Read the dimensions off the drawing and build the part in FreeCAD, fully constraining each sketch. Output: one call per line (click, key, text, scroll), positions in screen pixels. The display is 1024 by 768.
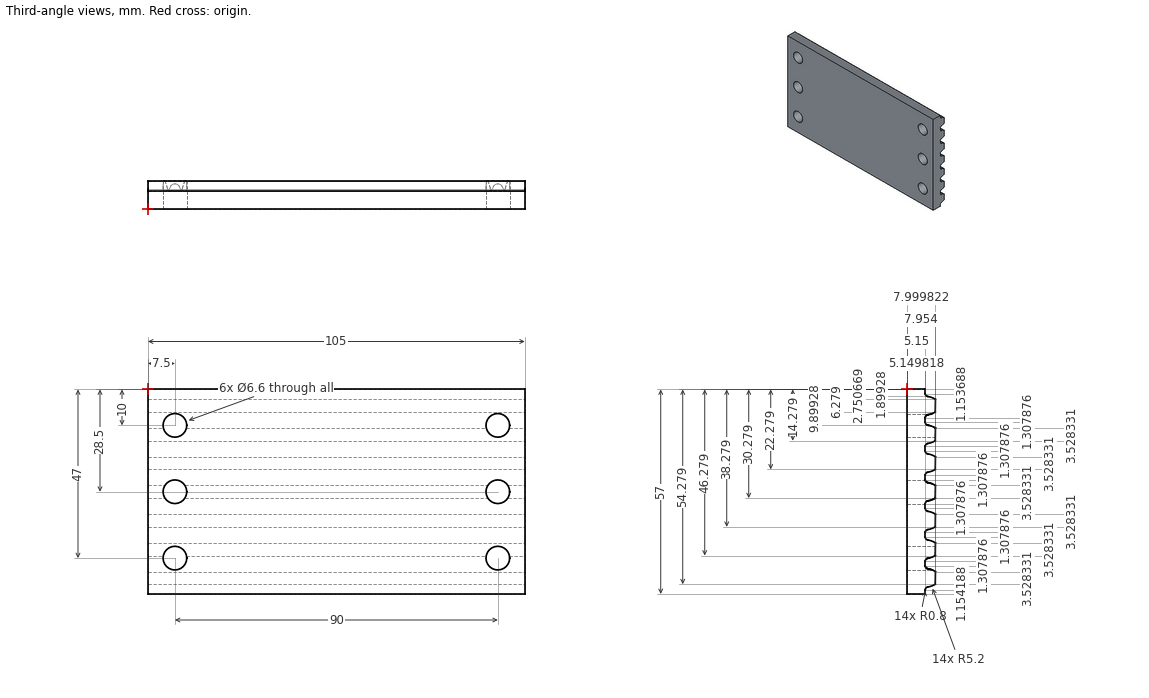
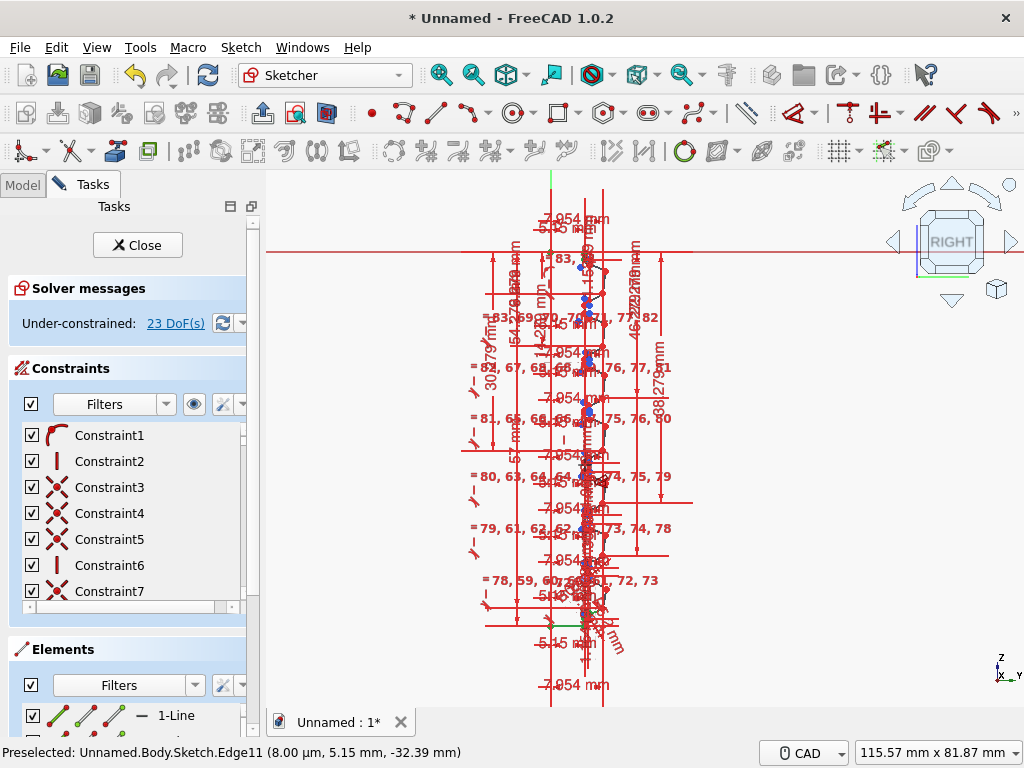
scroll(585, 413, up, 13)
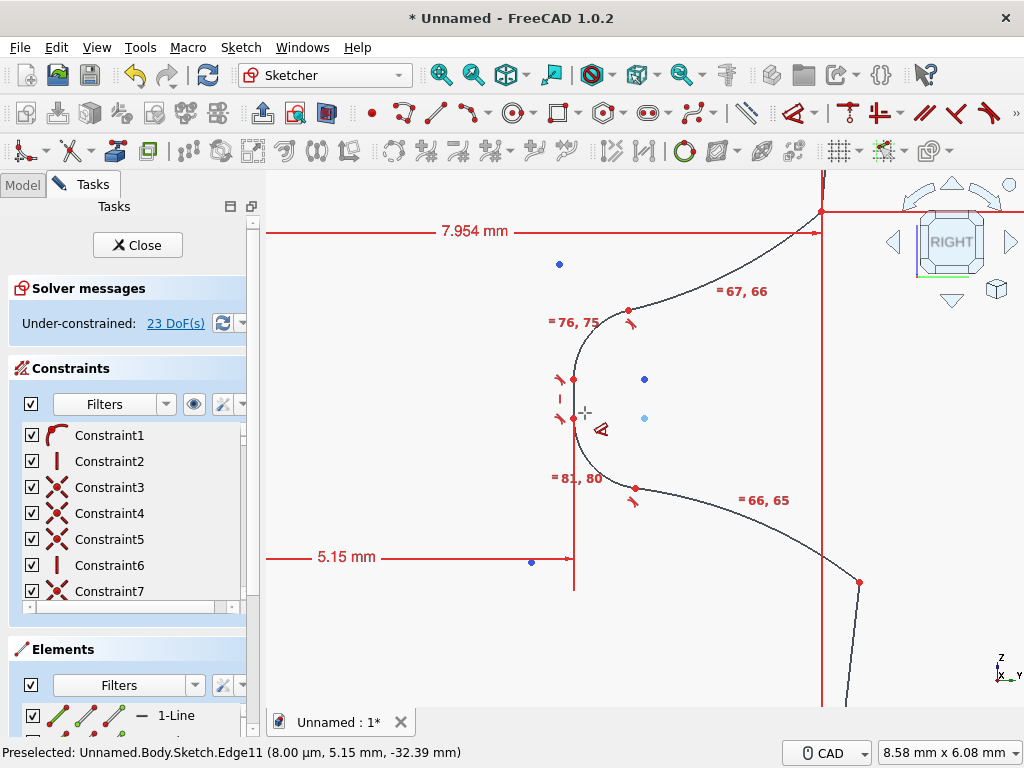
click(574, 403)
click(608, 399)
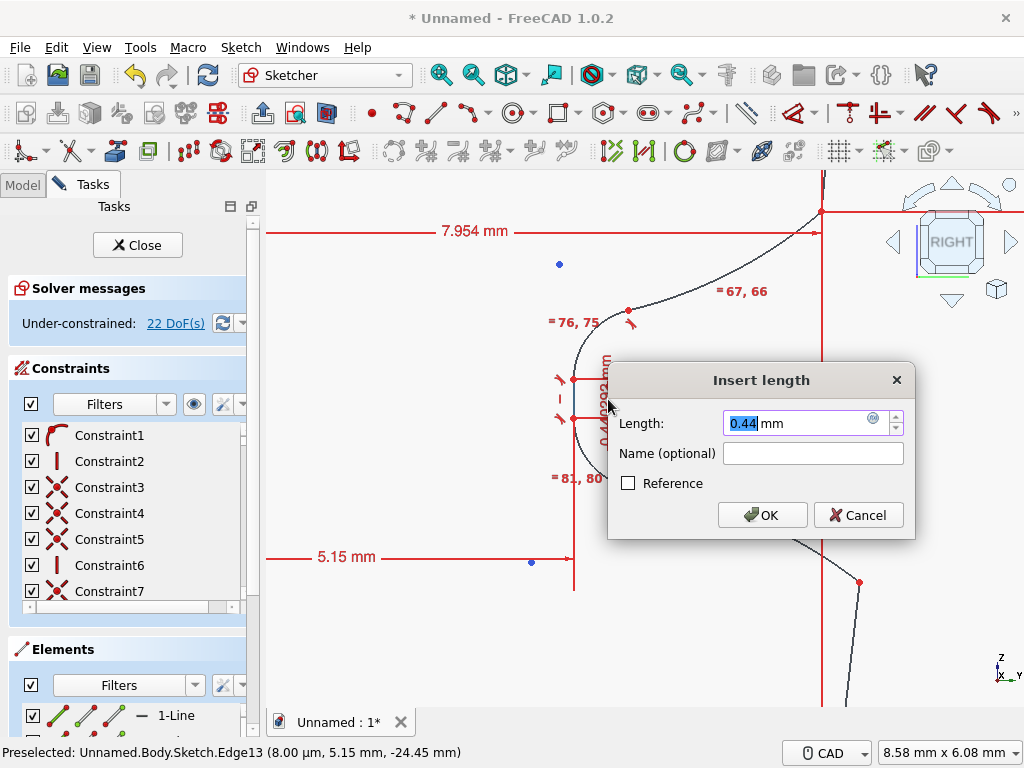
text(1.307876)
key(Return)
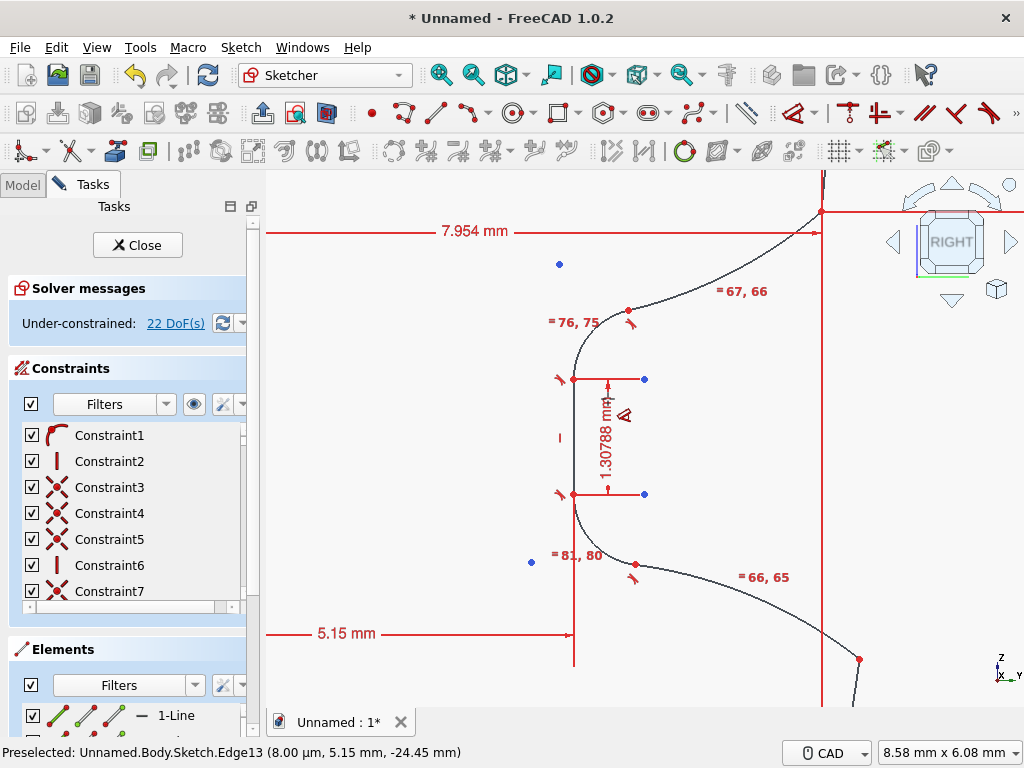
scroll(585, 413, down, 13)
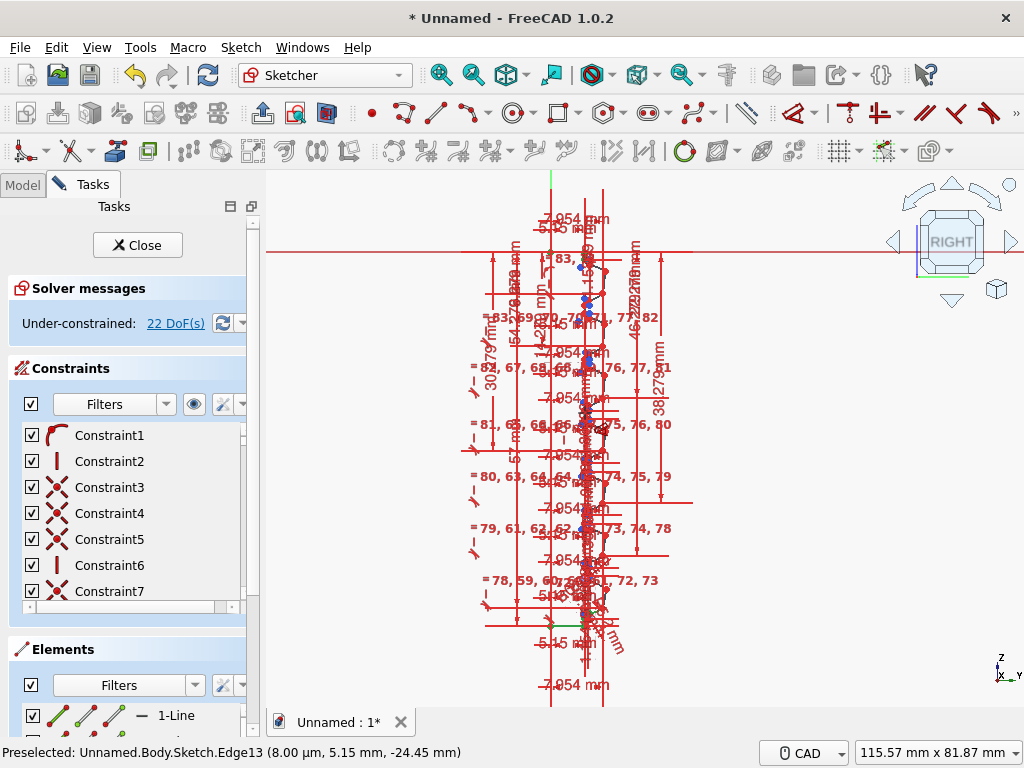
scroll(585, 362, up, 13)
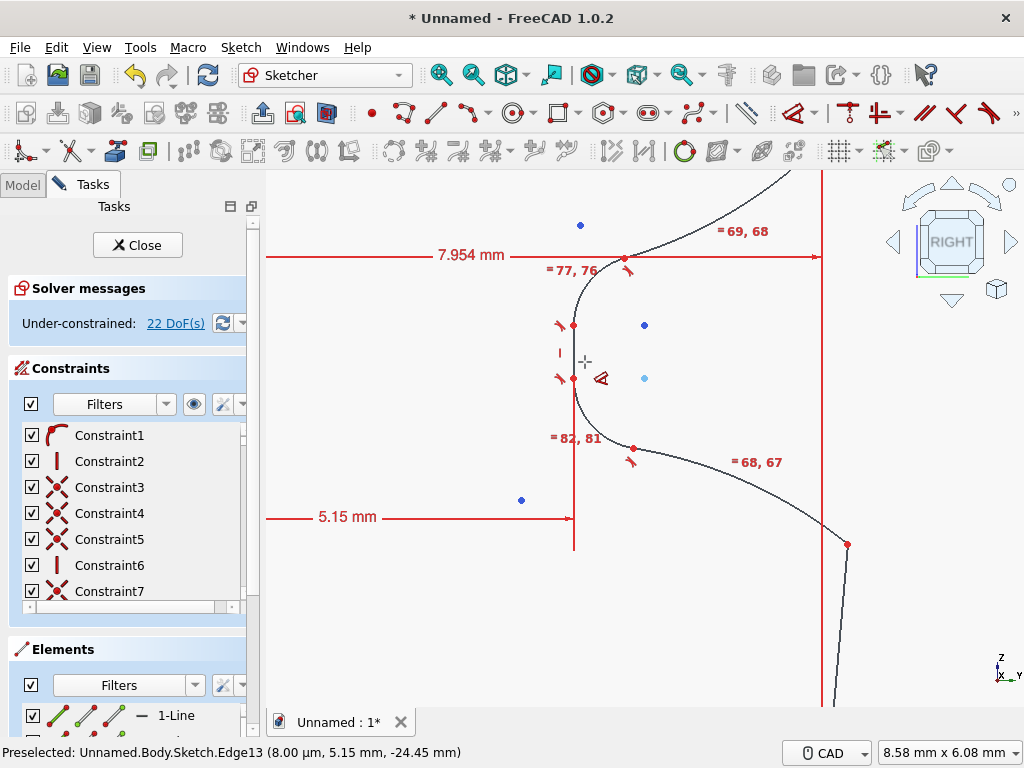
click(574, 363)
click(608, 352)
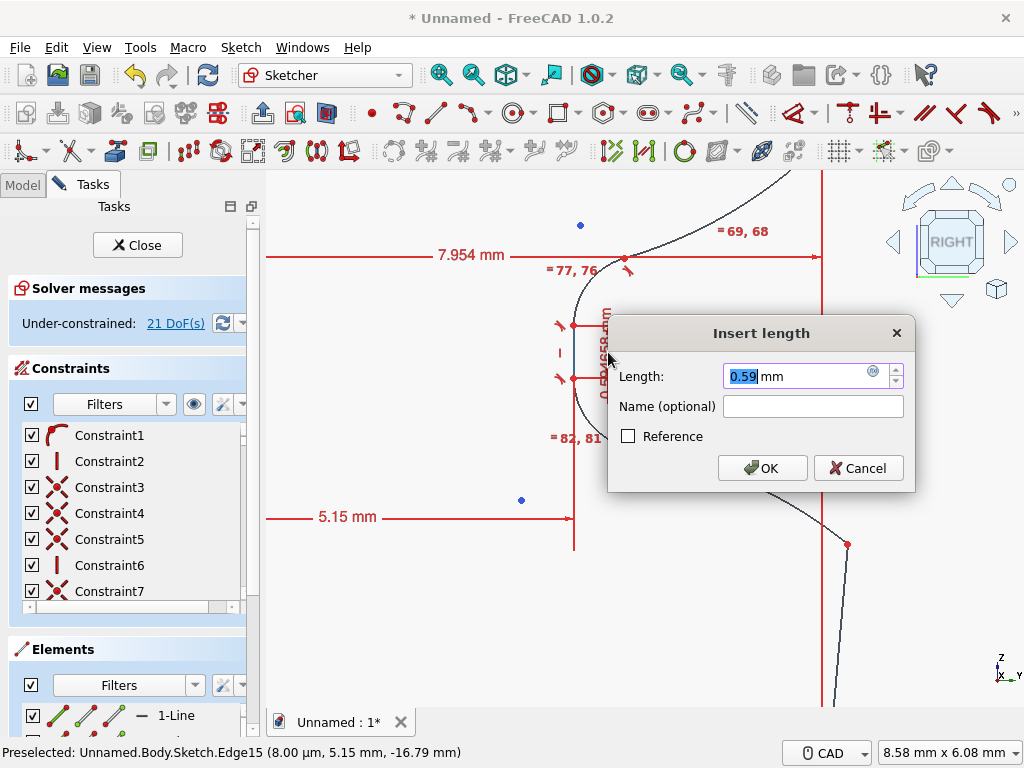
text(1.307876)
key(Return)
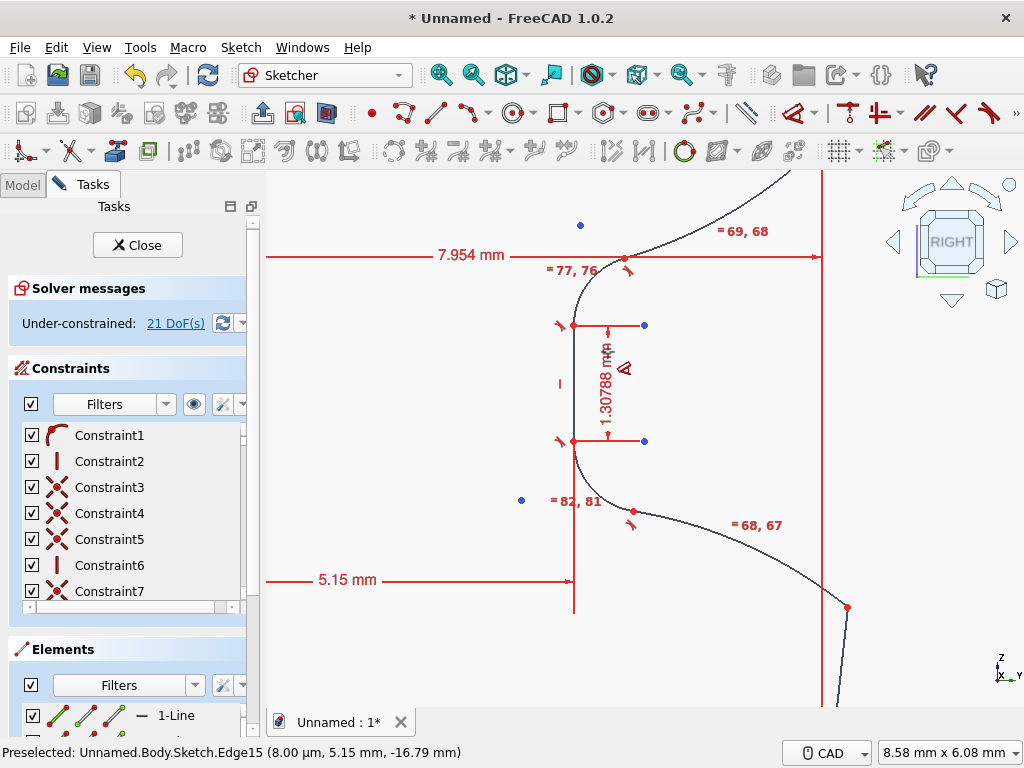
scroll(585, 362, down, 13)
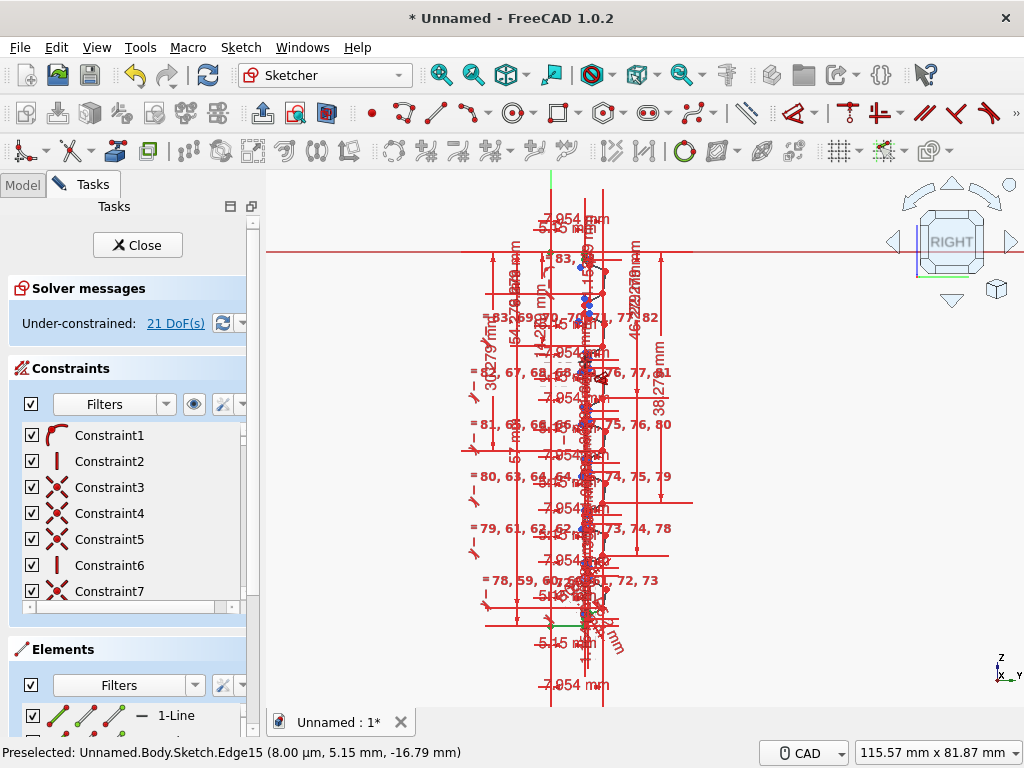
scroll(585, 311, up, 10)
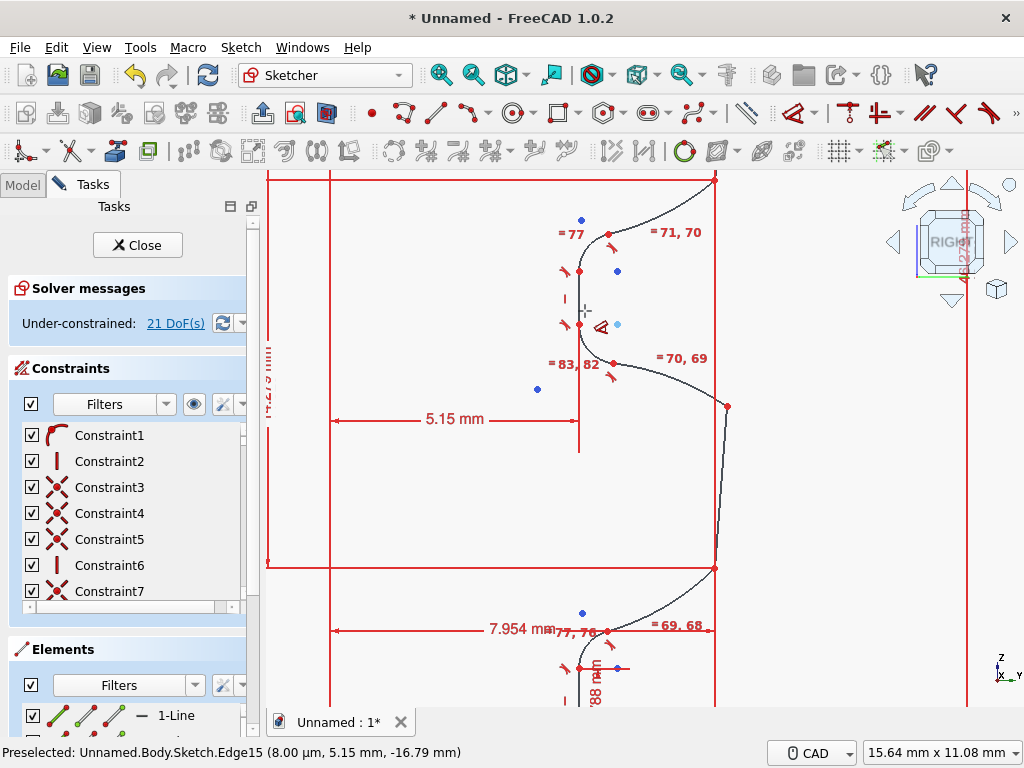
click(579, 309)
click(613, 298)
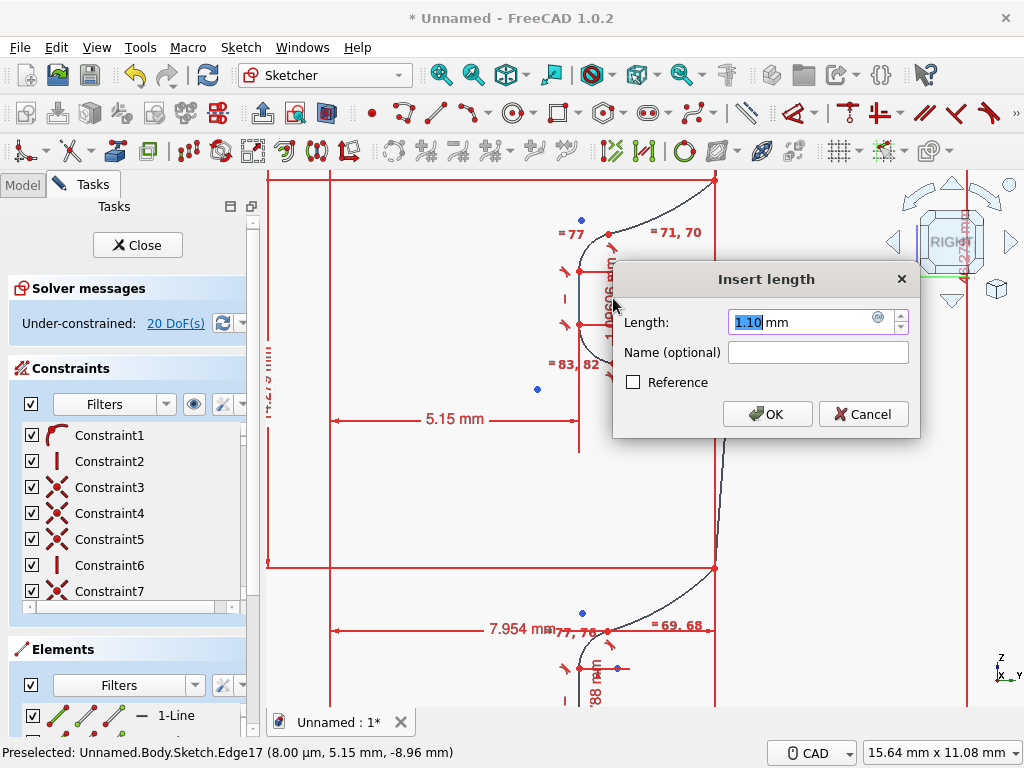
text(1.307876)
key(Return)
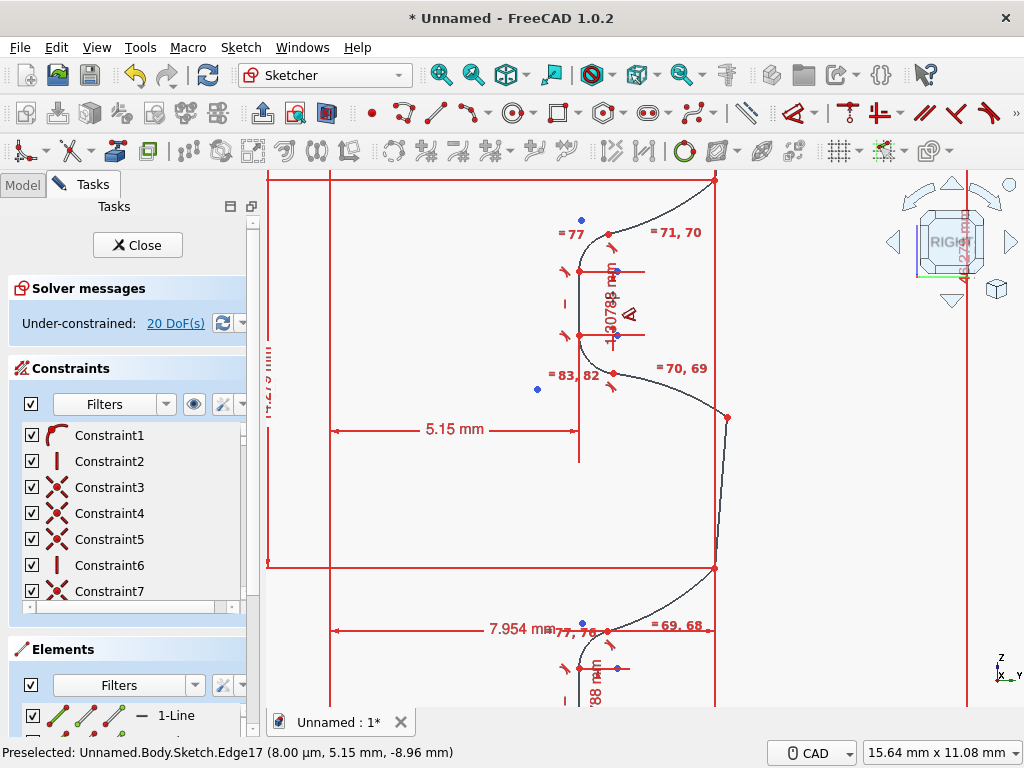
scroll(585, 310, down, 10)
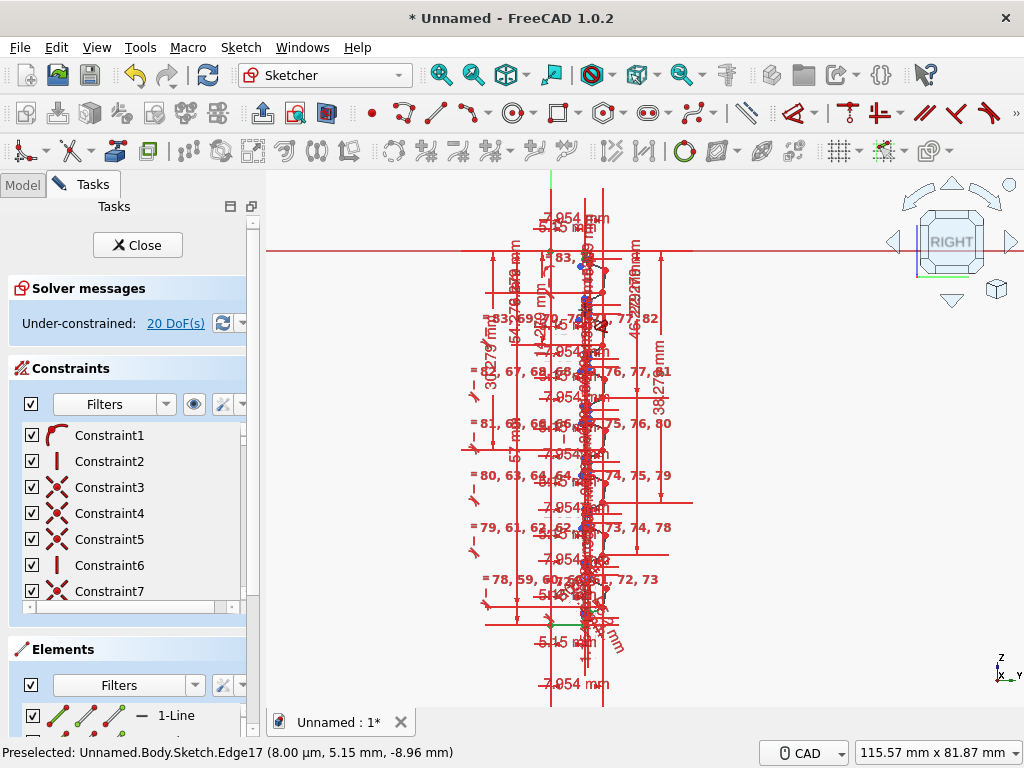
scroll(579, 321, up, 2)